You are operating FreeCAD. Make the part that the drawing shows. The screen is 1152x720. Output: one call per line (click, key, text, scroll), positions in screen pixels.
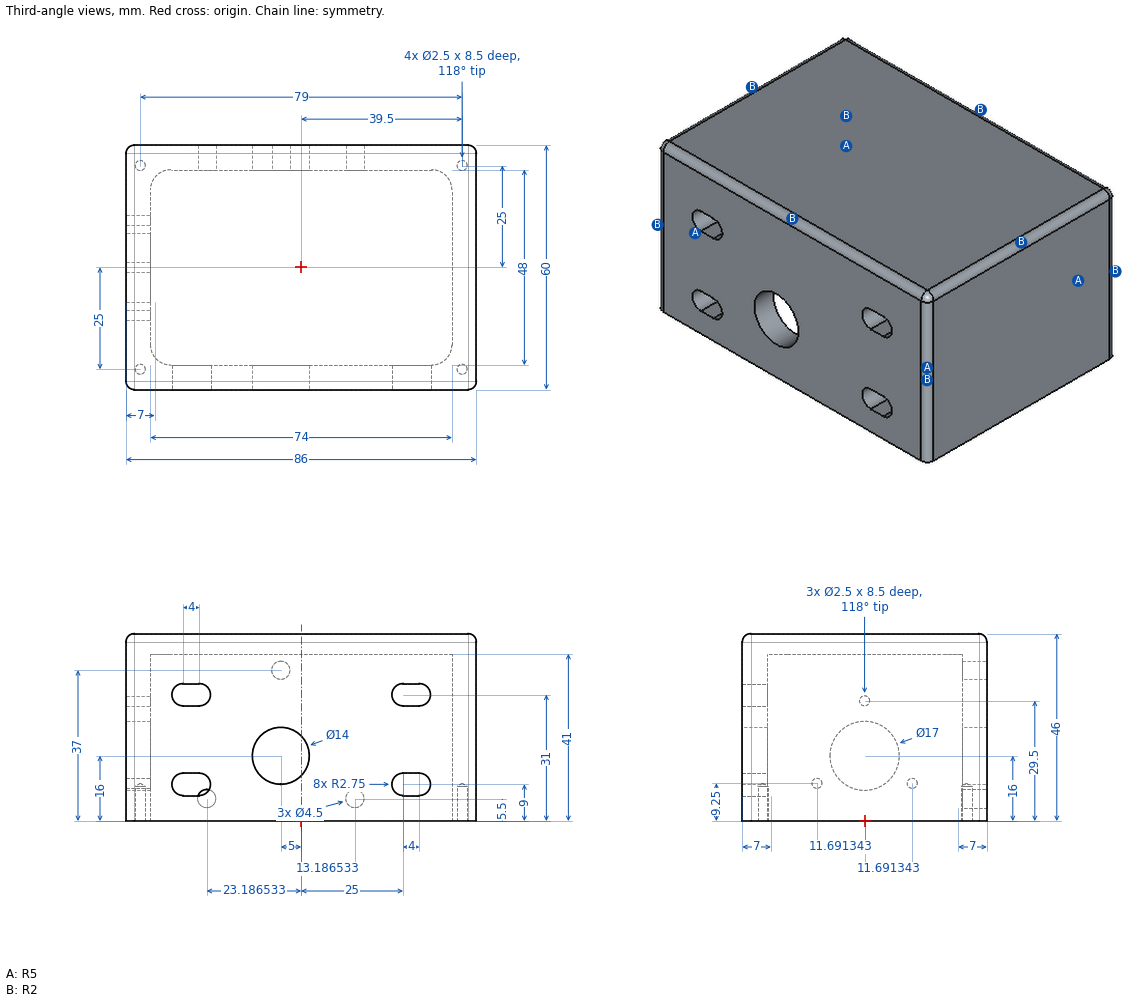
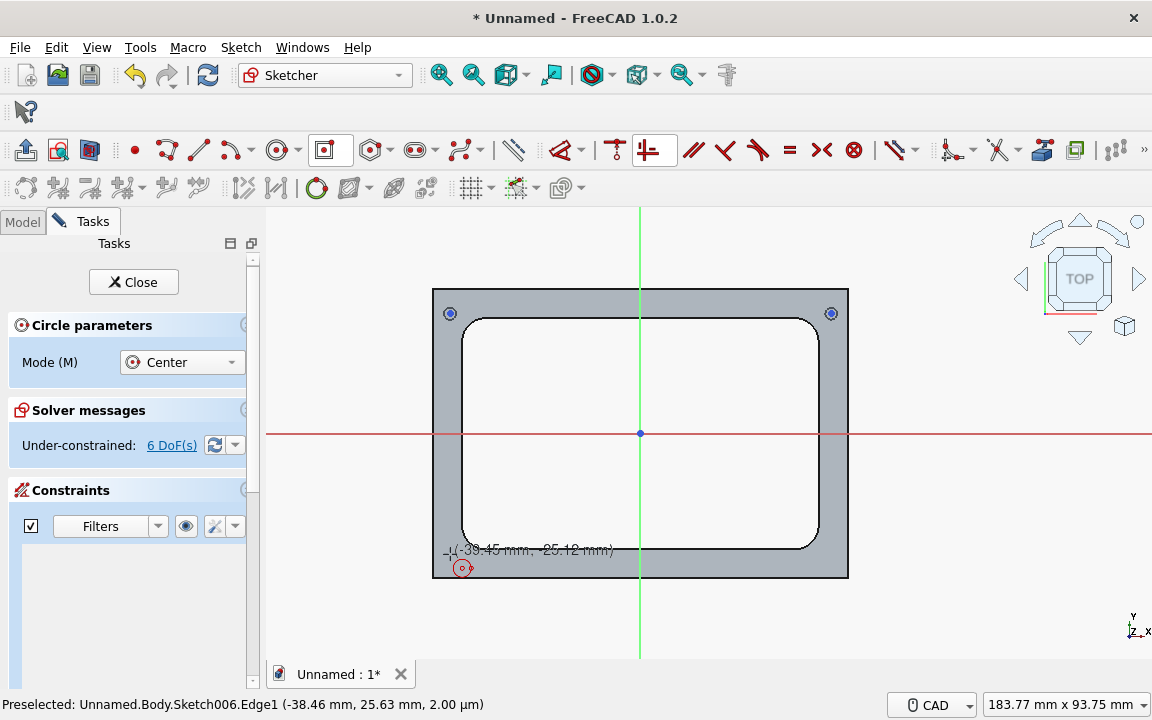
click(450, 554)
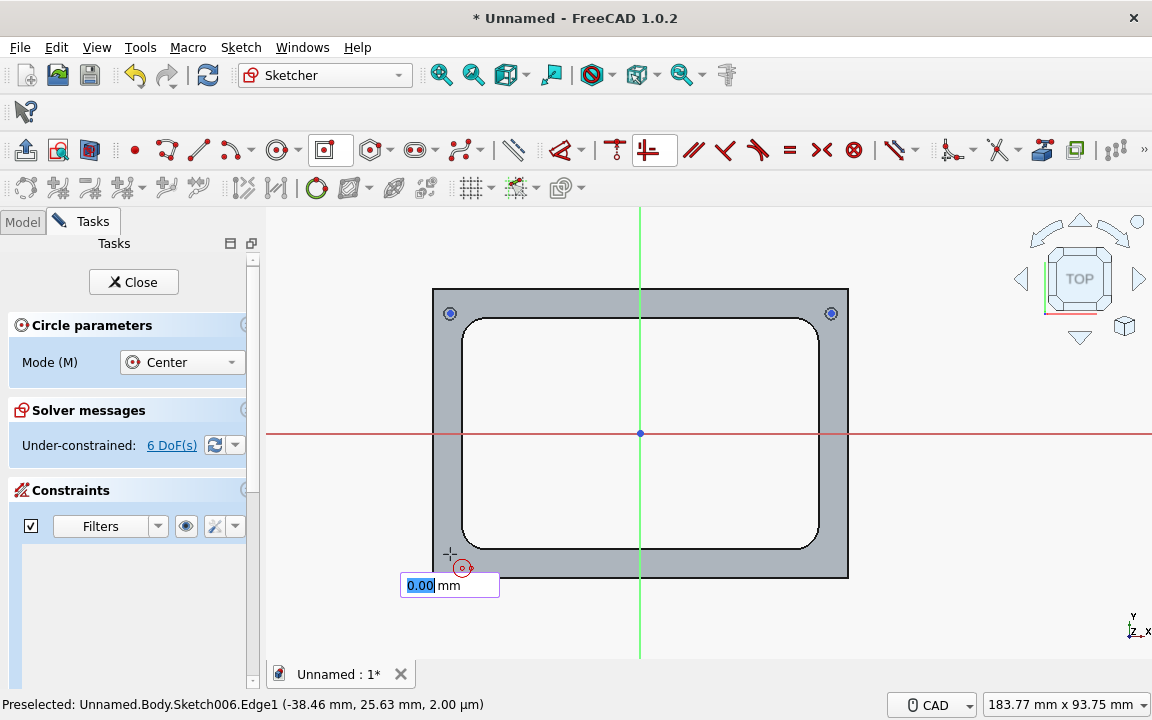
scroll(454, 550, up, 5)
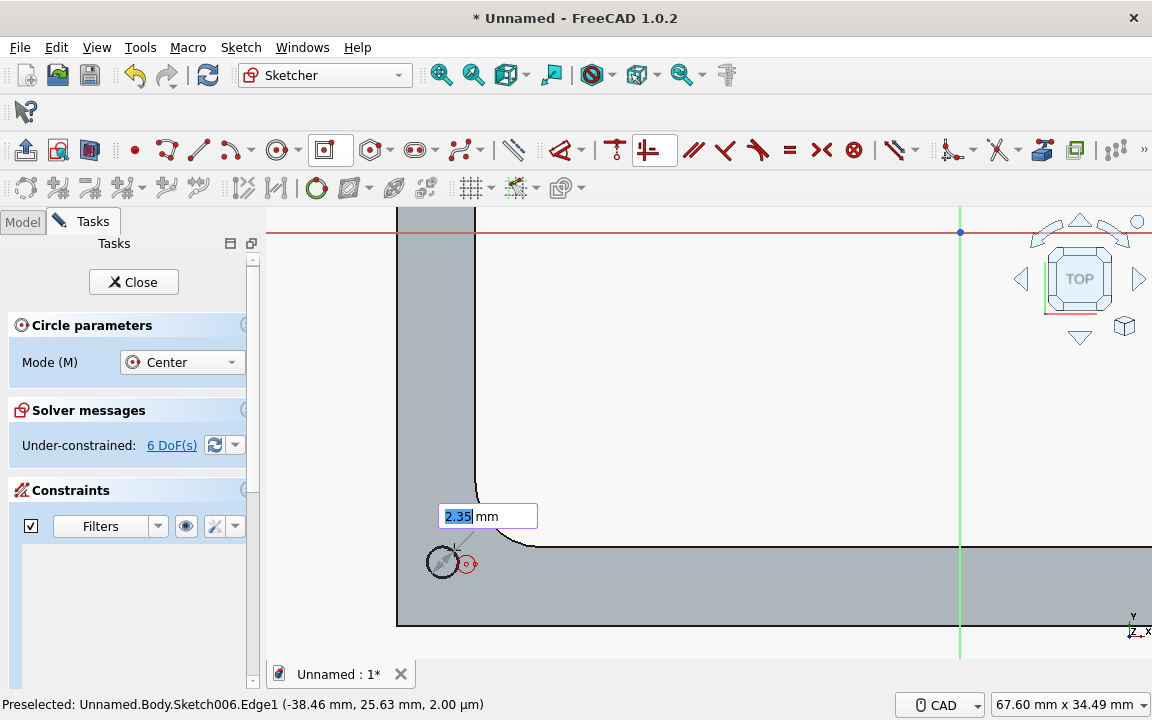
click(454, 549)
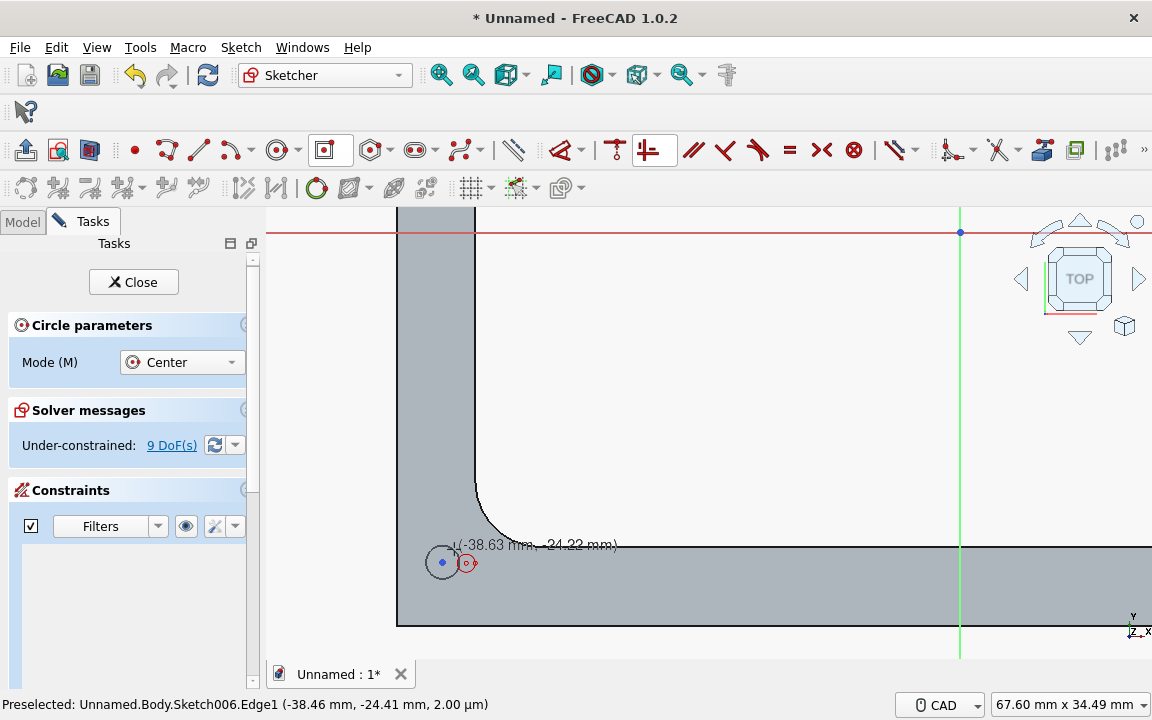
scroll(454, 550, down, 5)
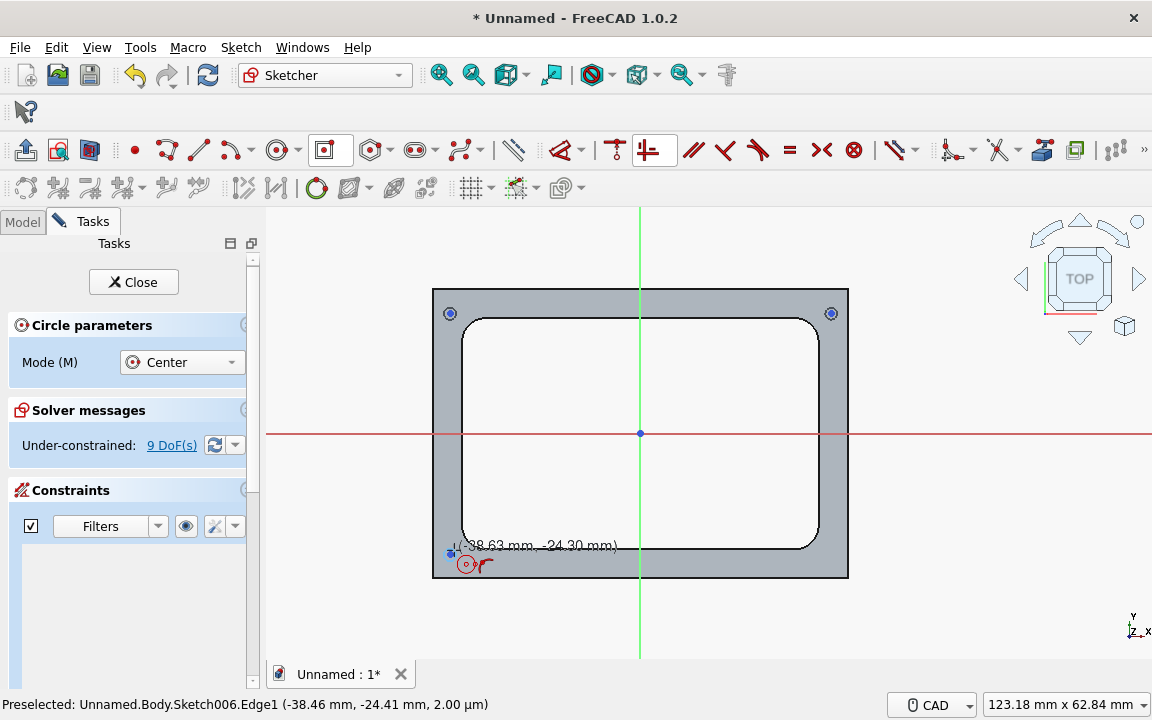
scroll(831, 554, up, 7)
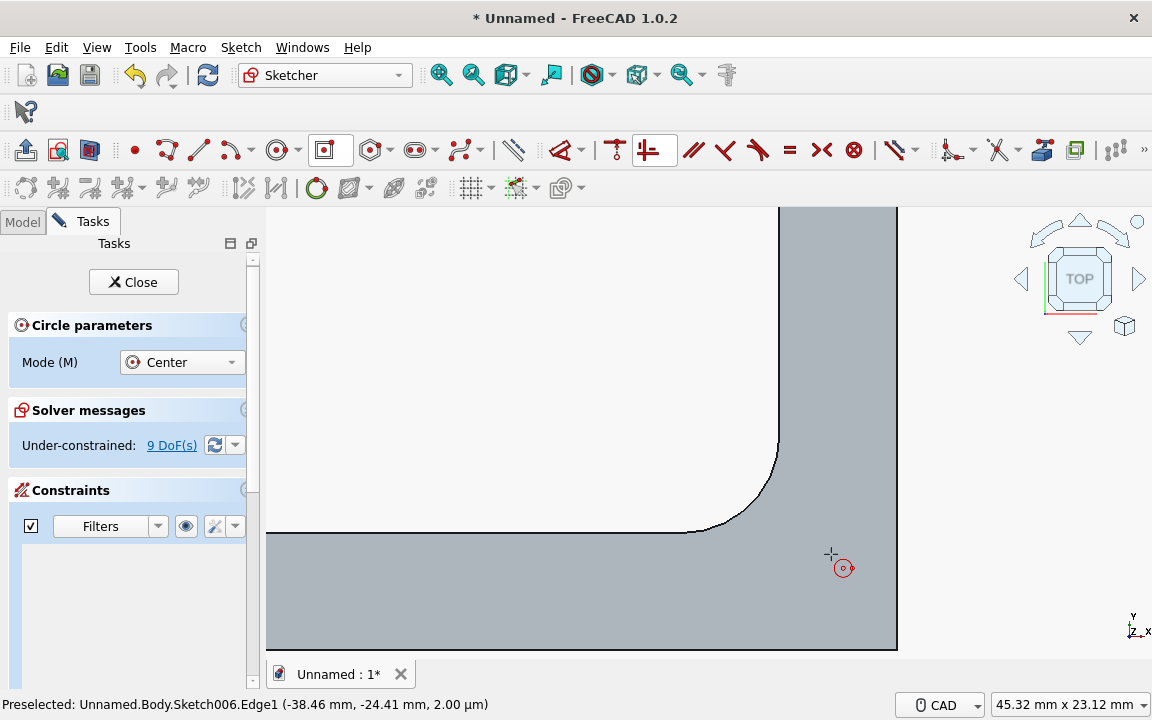
scroll(832, 554, down, 7)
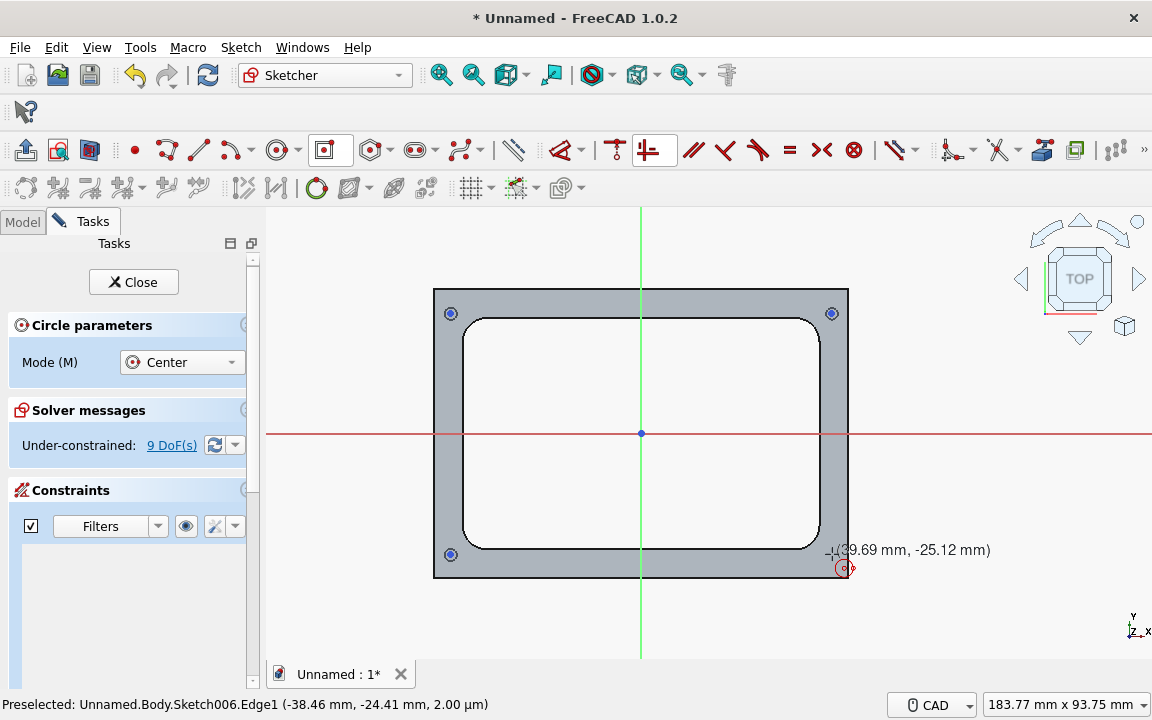
click(832, 554)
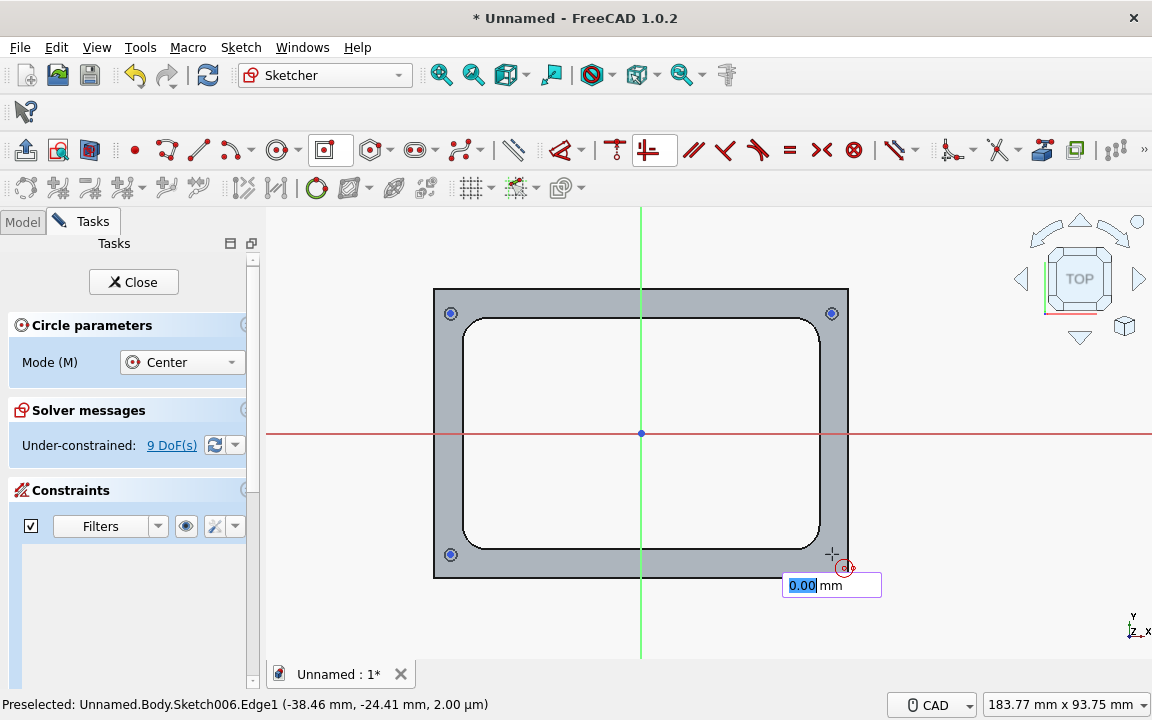
scroll(836, 550, up, 5)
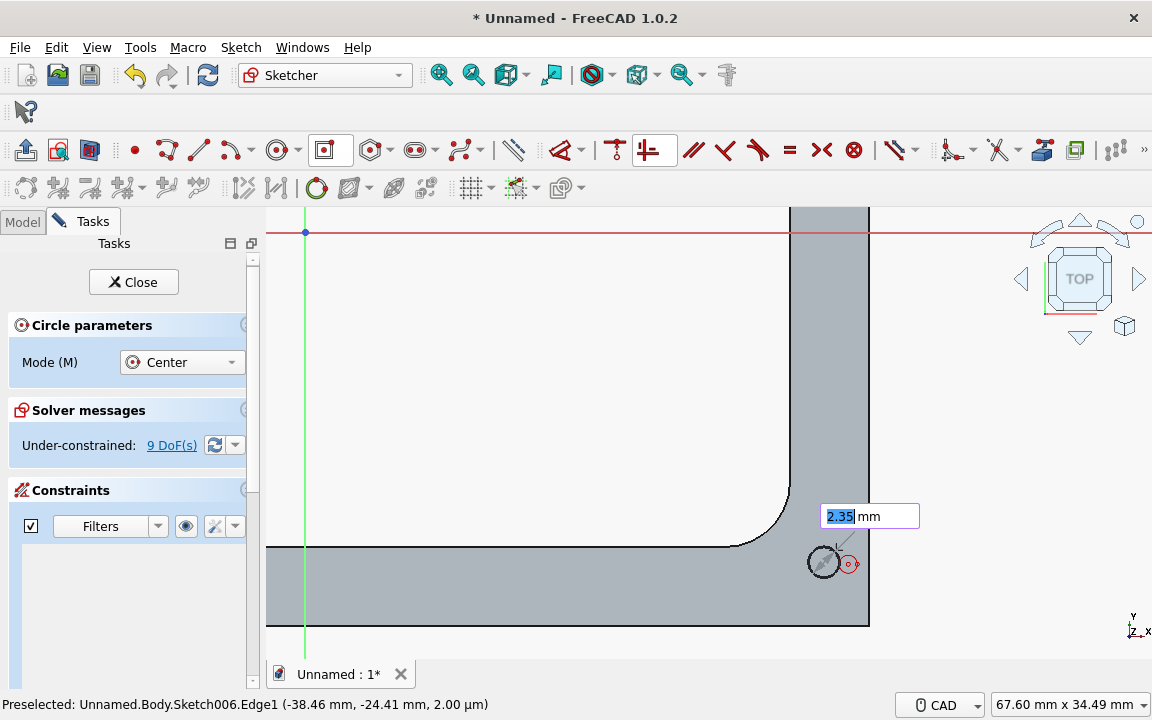
click(834, 549)
key(Escape)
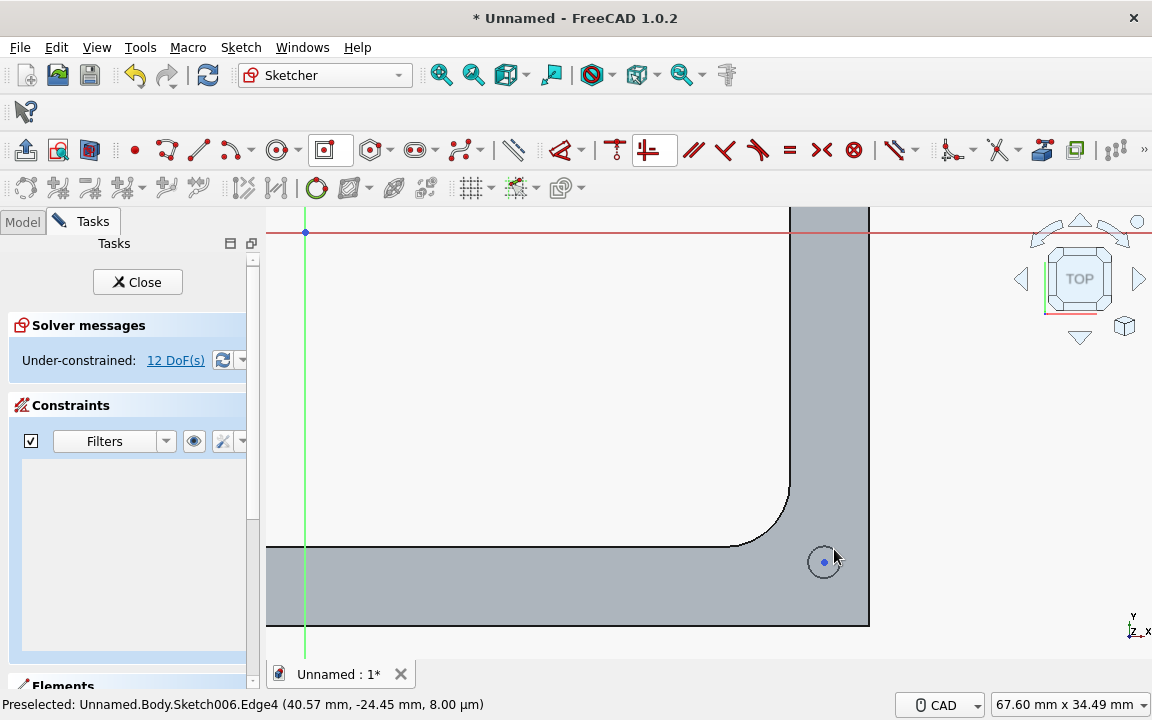
scroll(836, 550, down, 5)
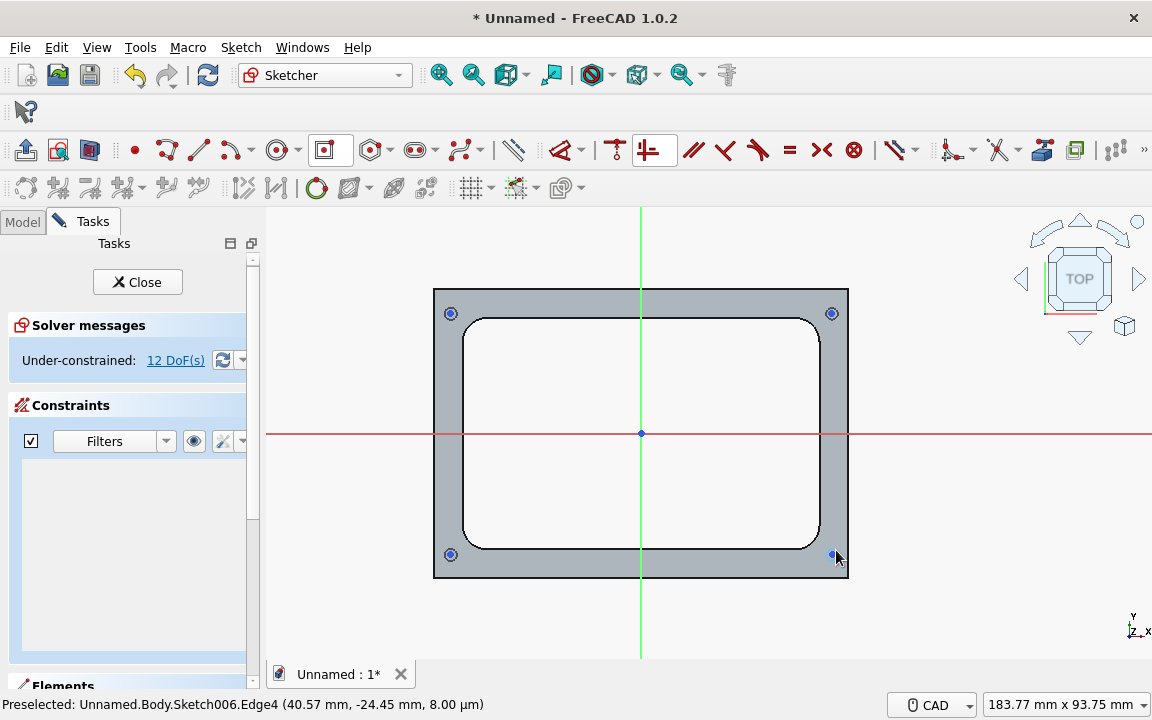
scroll(836, 310, up, 5)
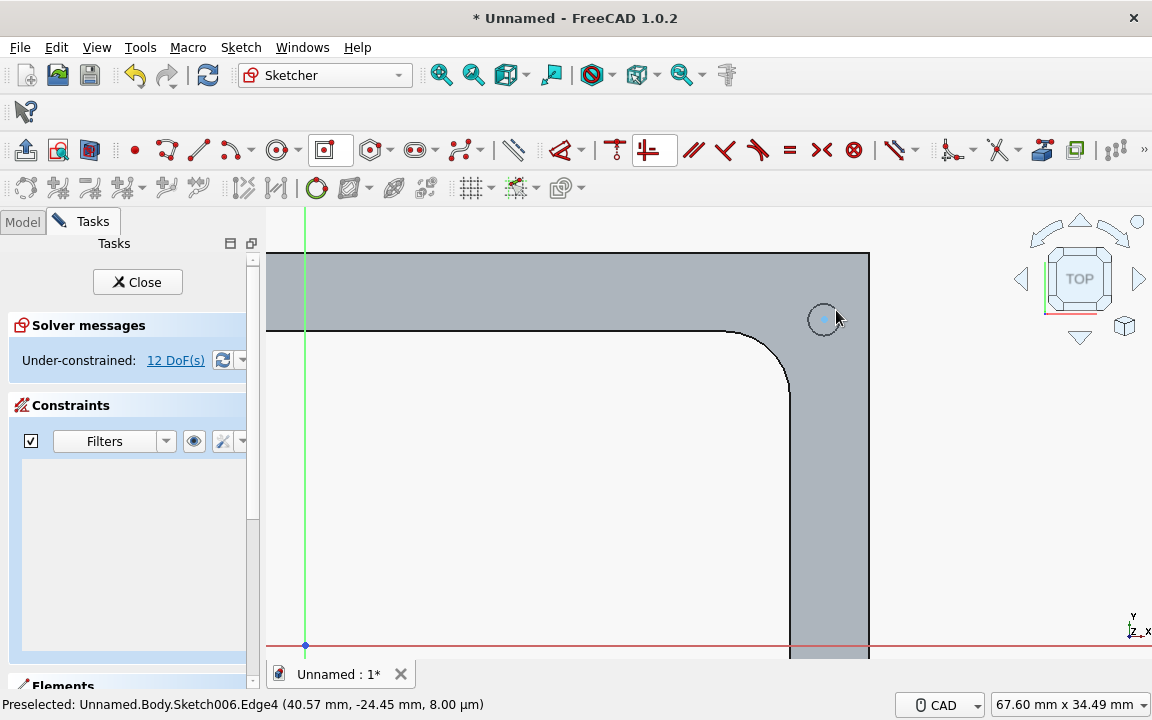
click(835, 309)